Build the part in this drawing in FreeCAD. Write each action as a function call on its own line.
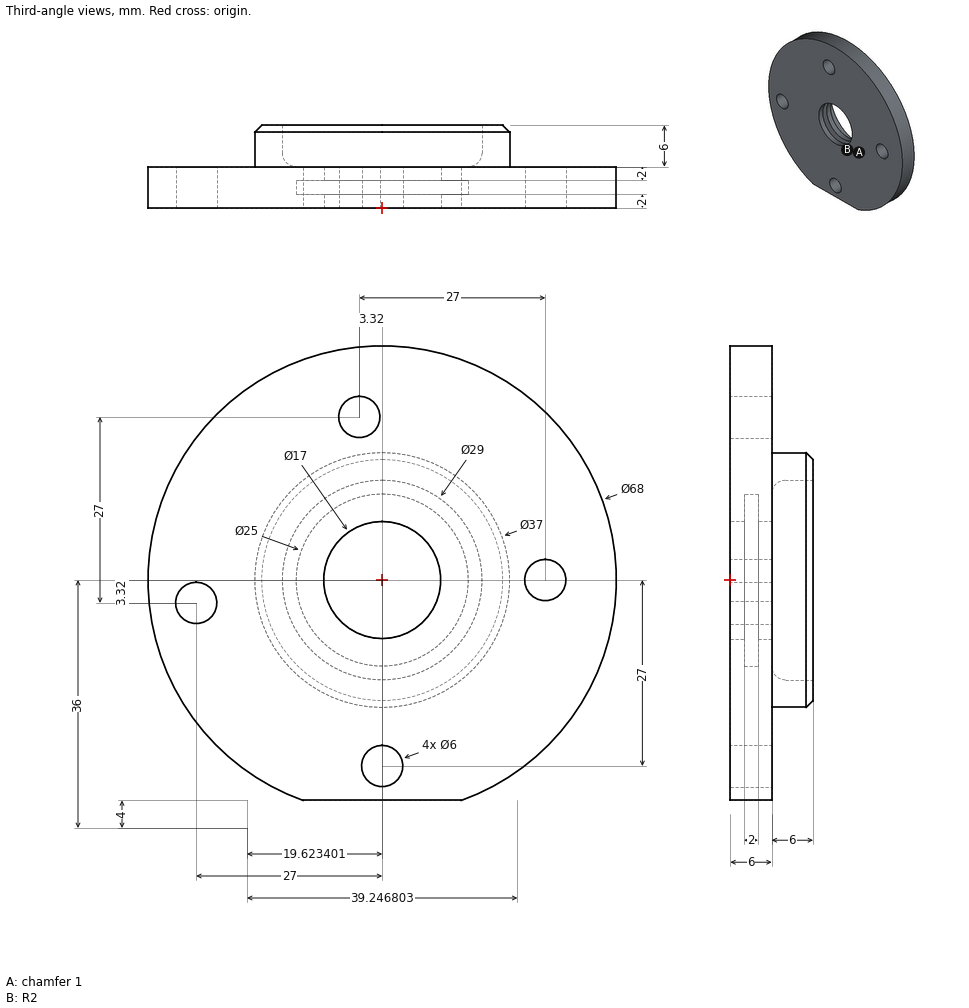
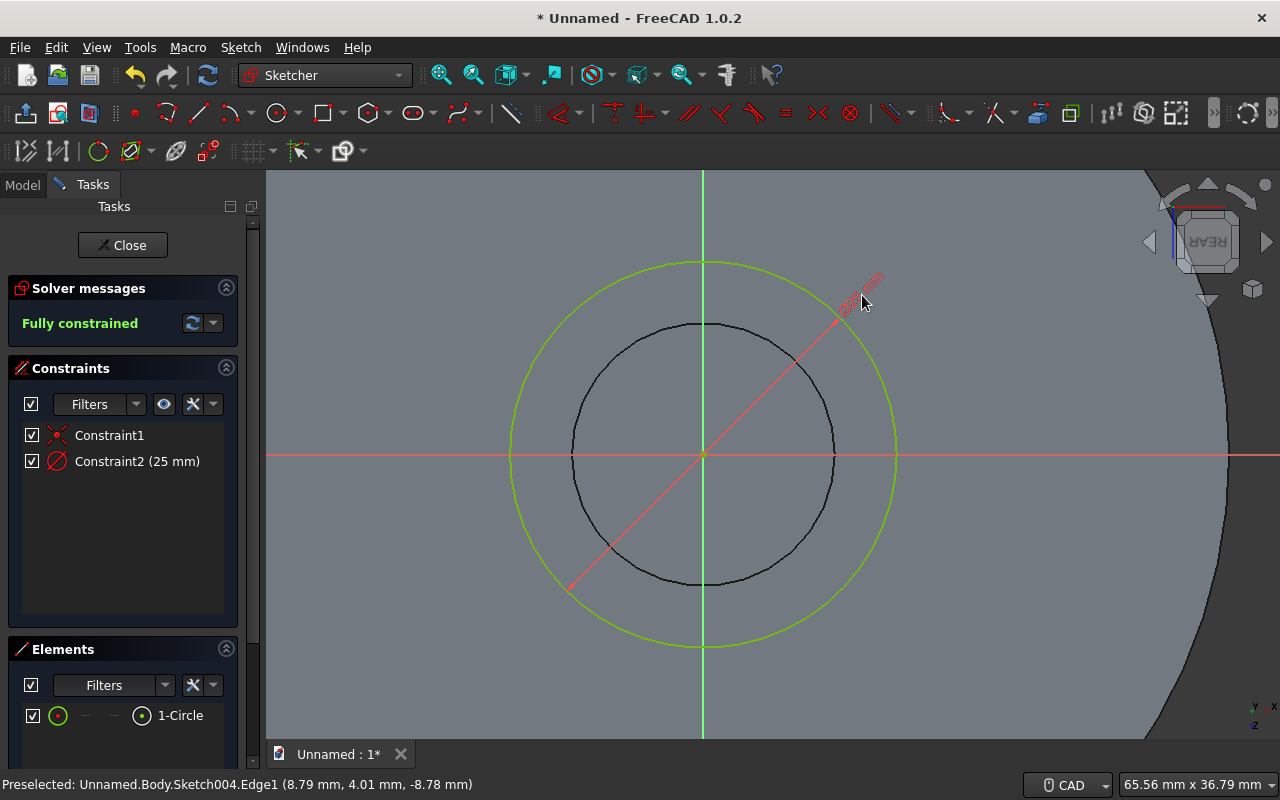
click(123, 245)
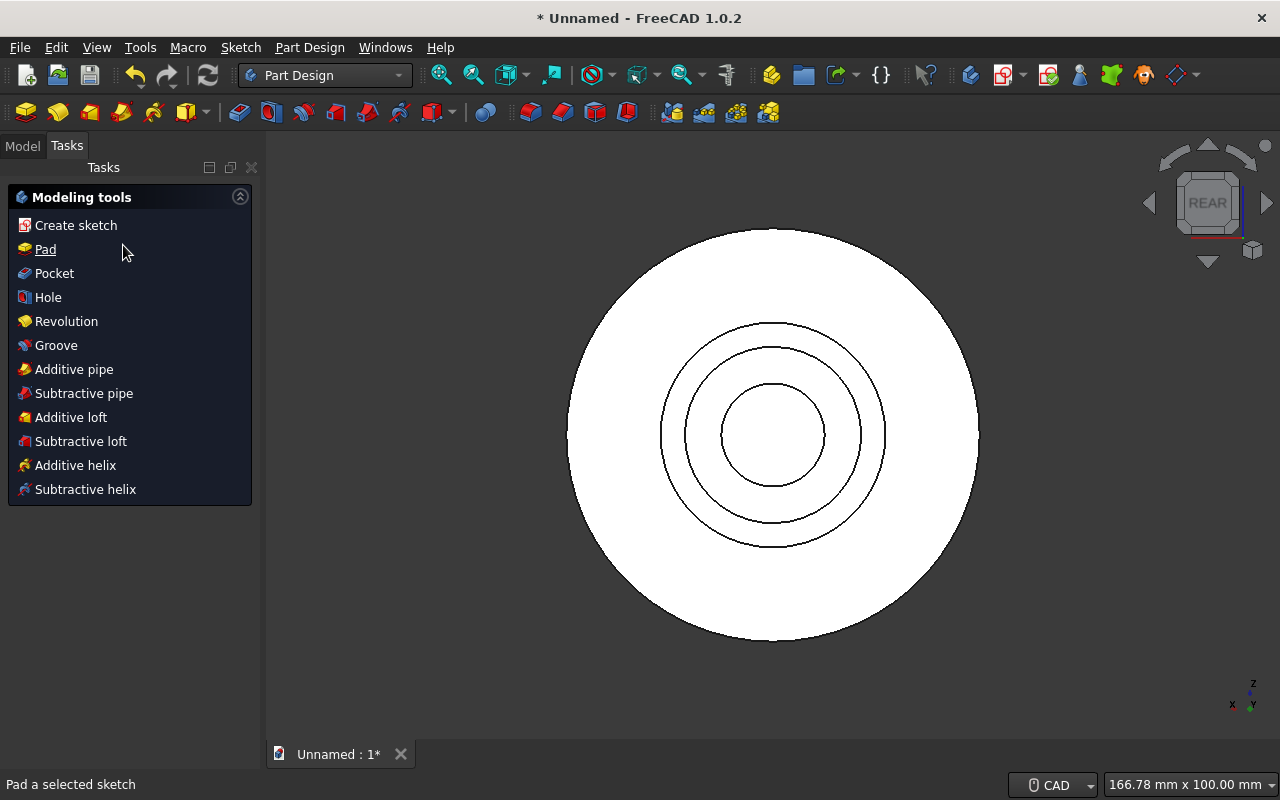
click(240, 112)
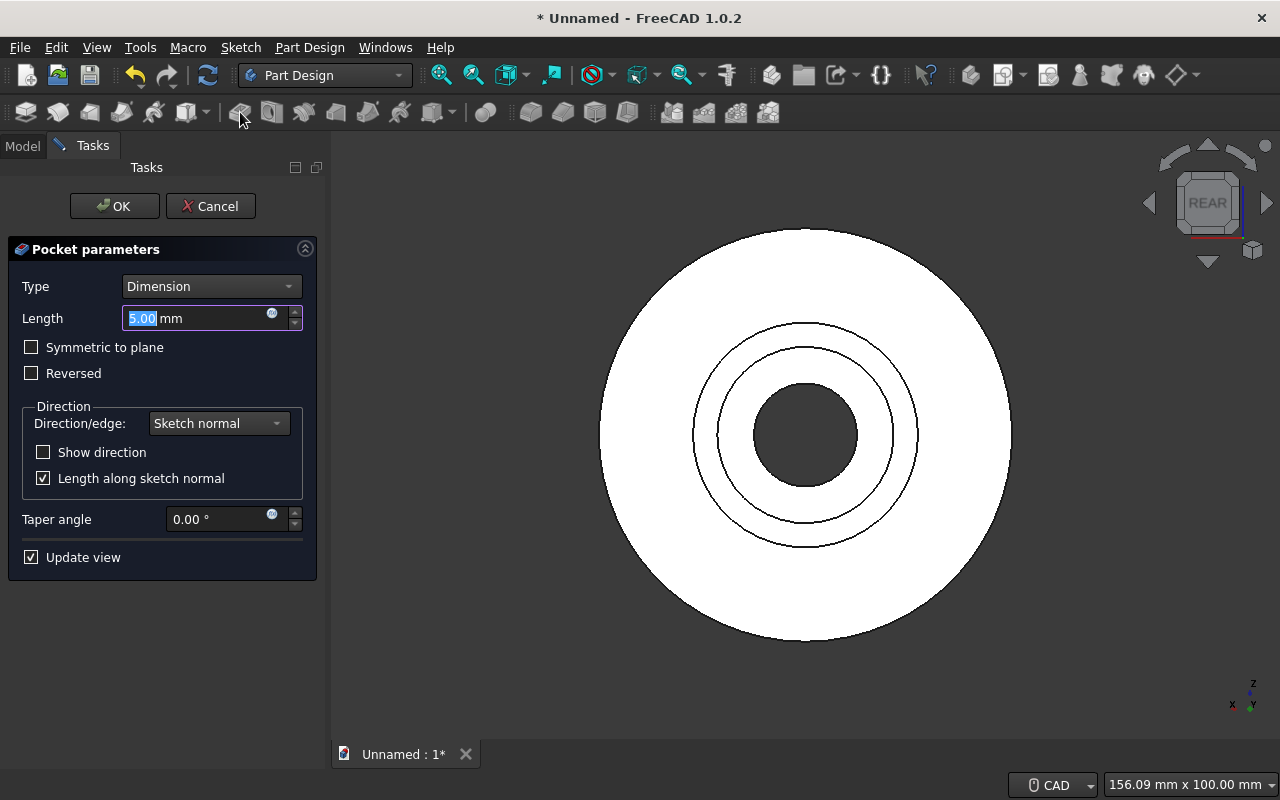
text(2)
key(Tab)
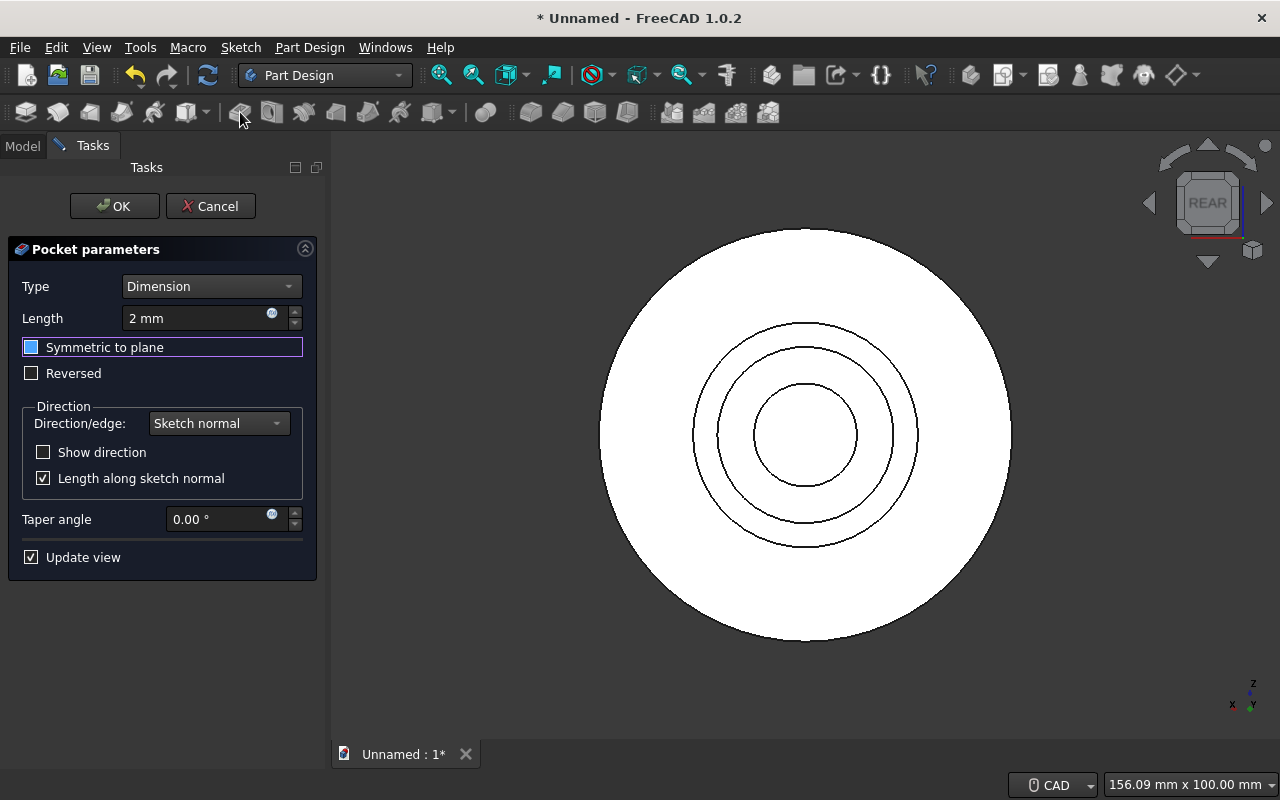
click(115, 206)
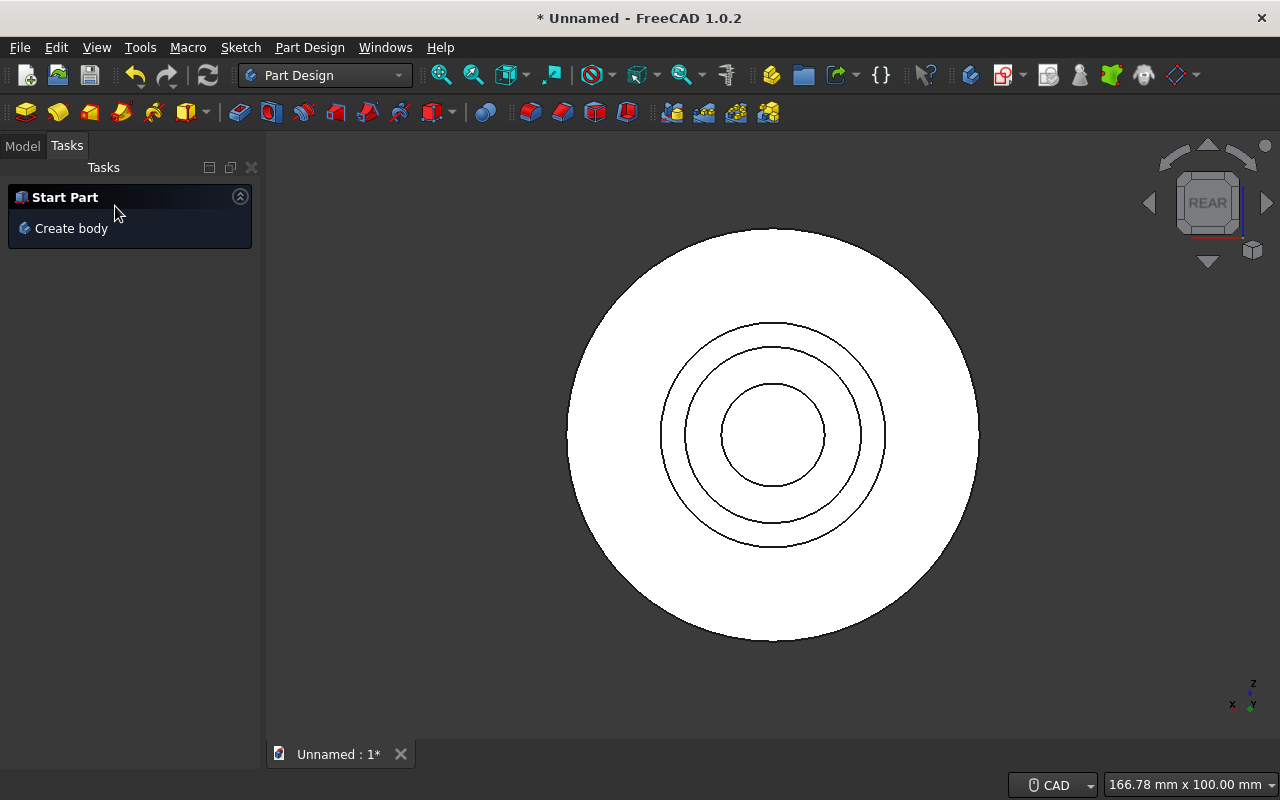
click(773, 434)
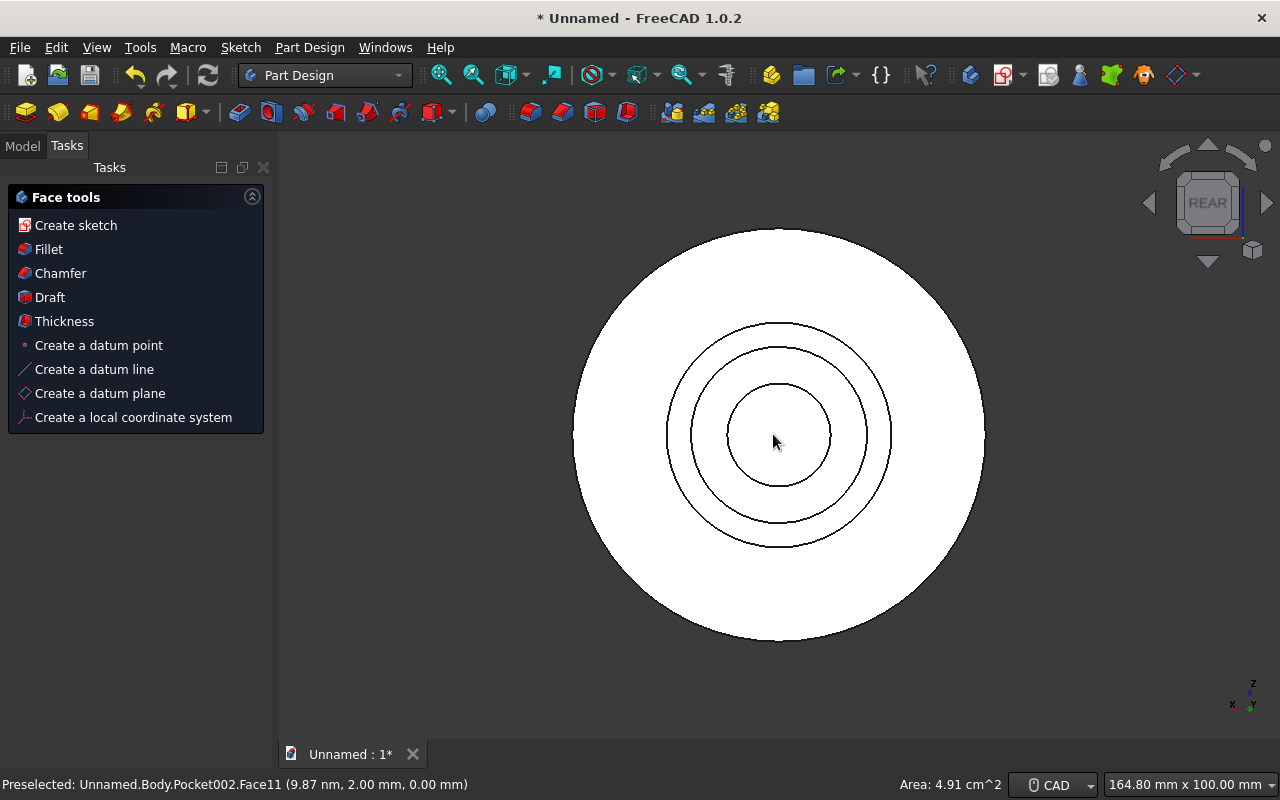
click(1004, 76)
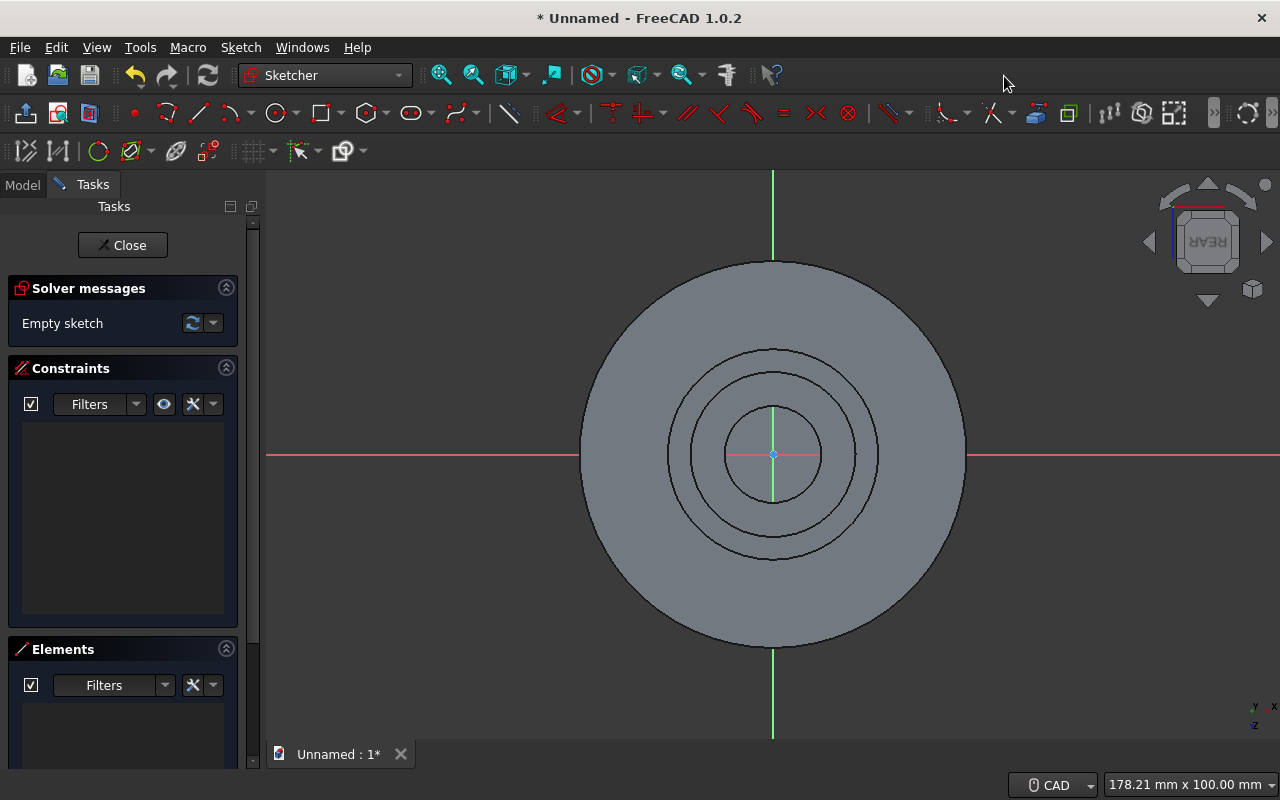
scroll(795, 454, up, 7)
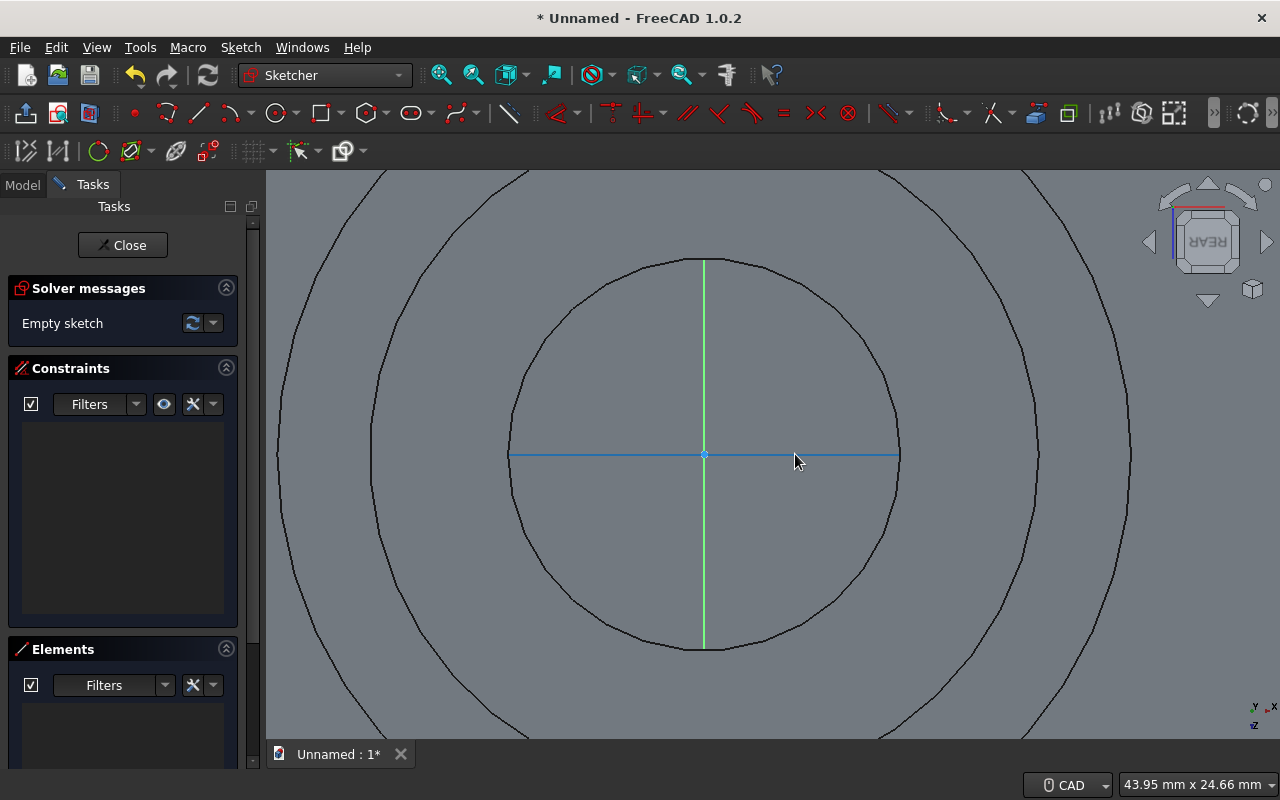
click(276, 114)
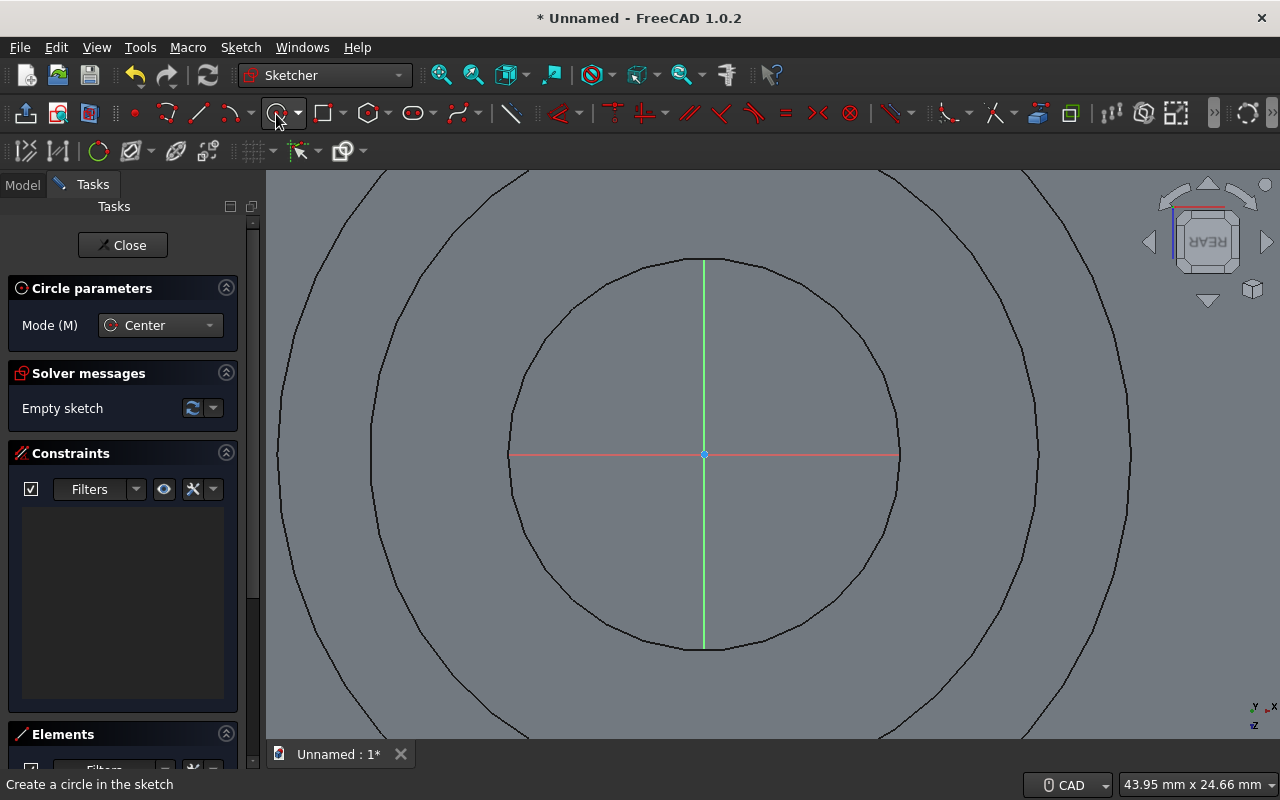
click(704, 454)
click(843, 316)
key(Escape)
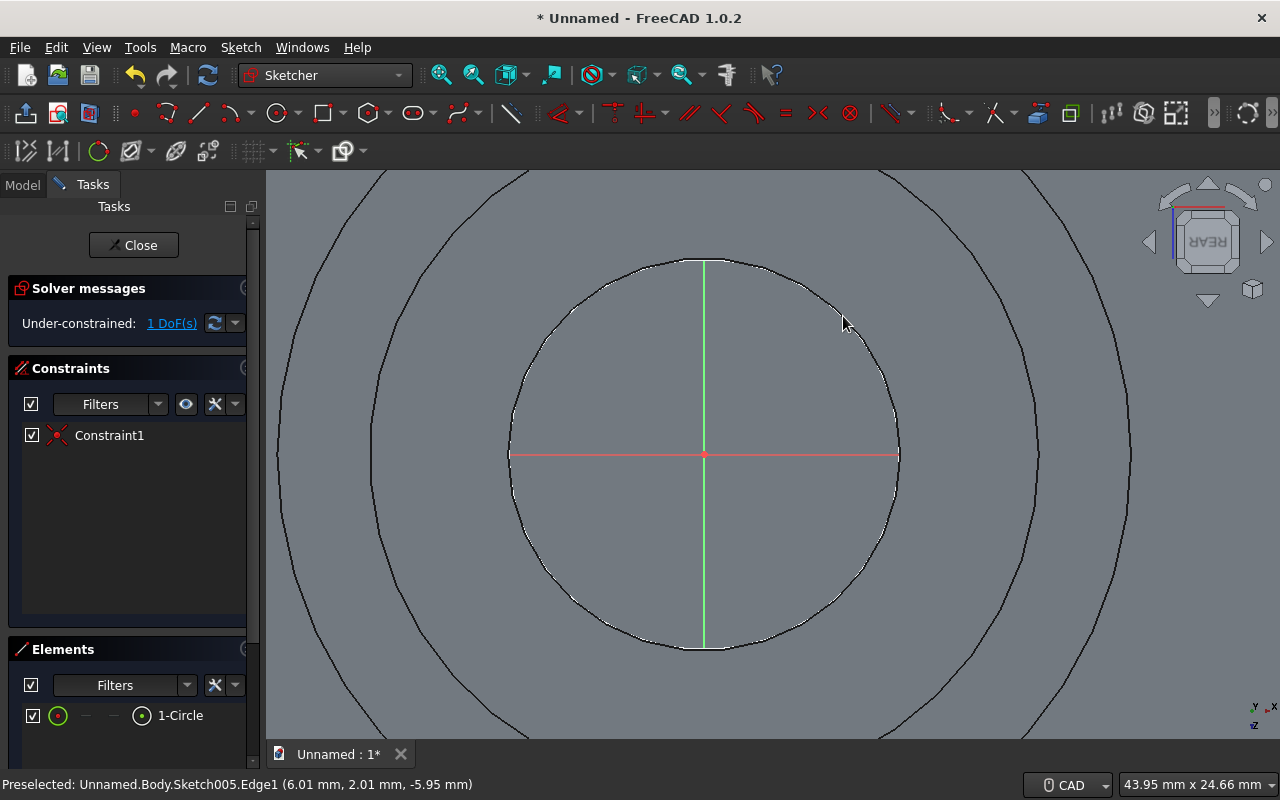
click(558, 114)